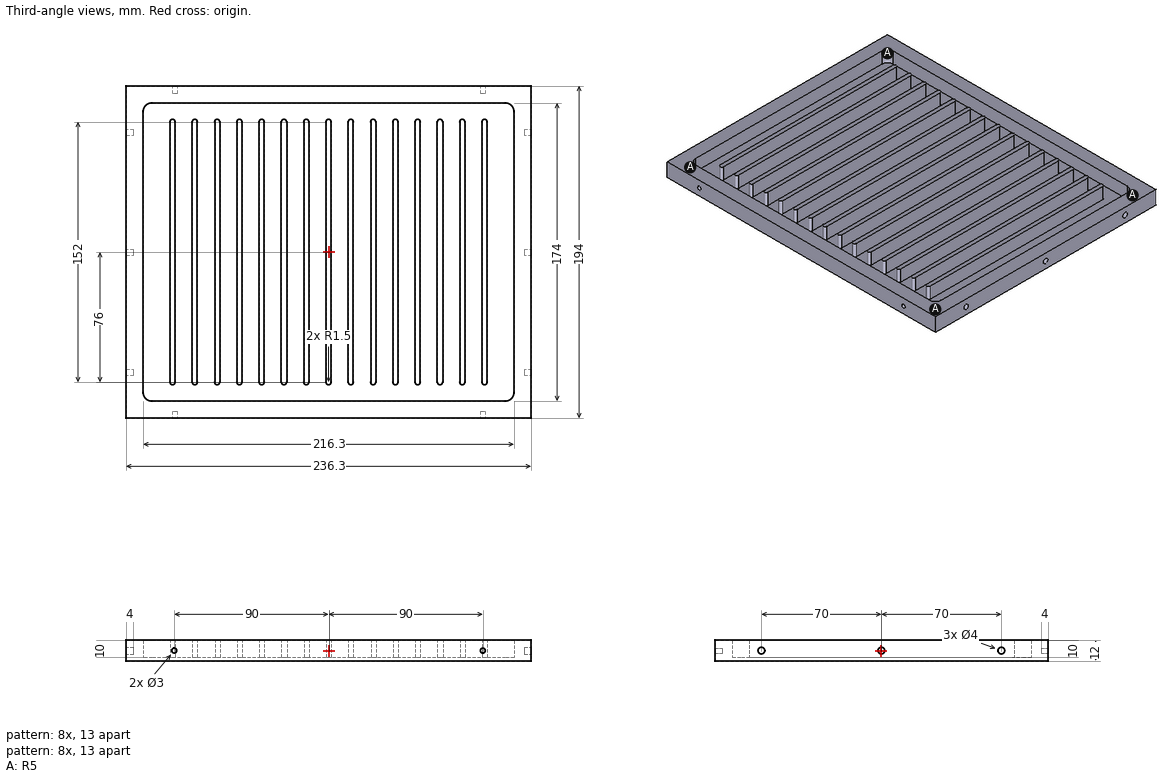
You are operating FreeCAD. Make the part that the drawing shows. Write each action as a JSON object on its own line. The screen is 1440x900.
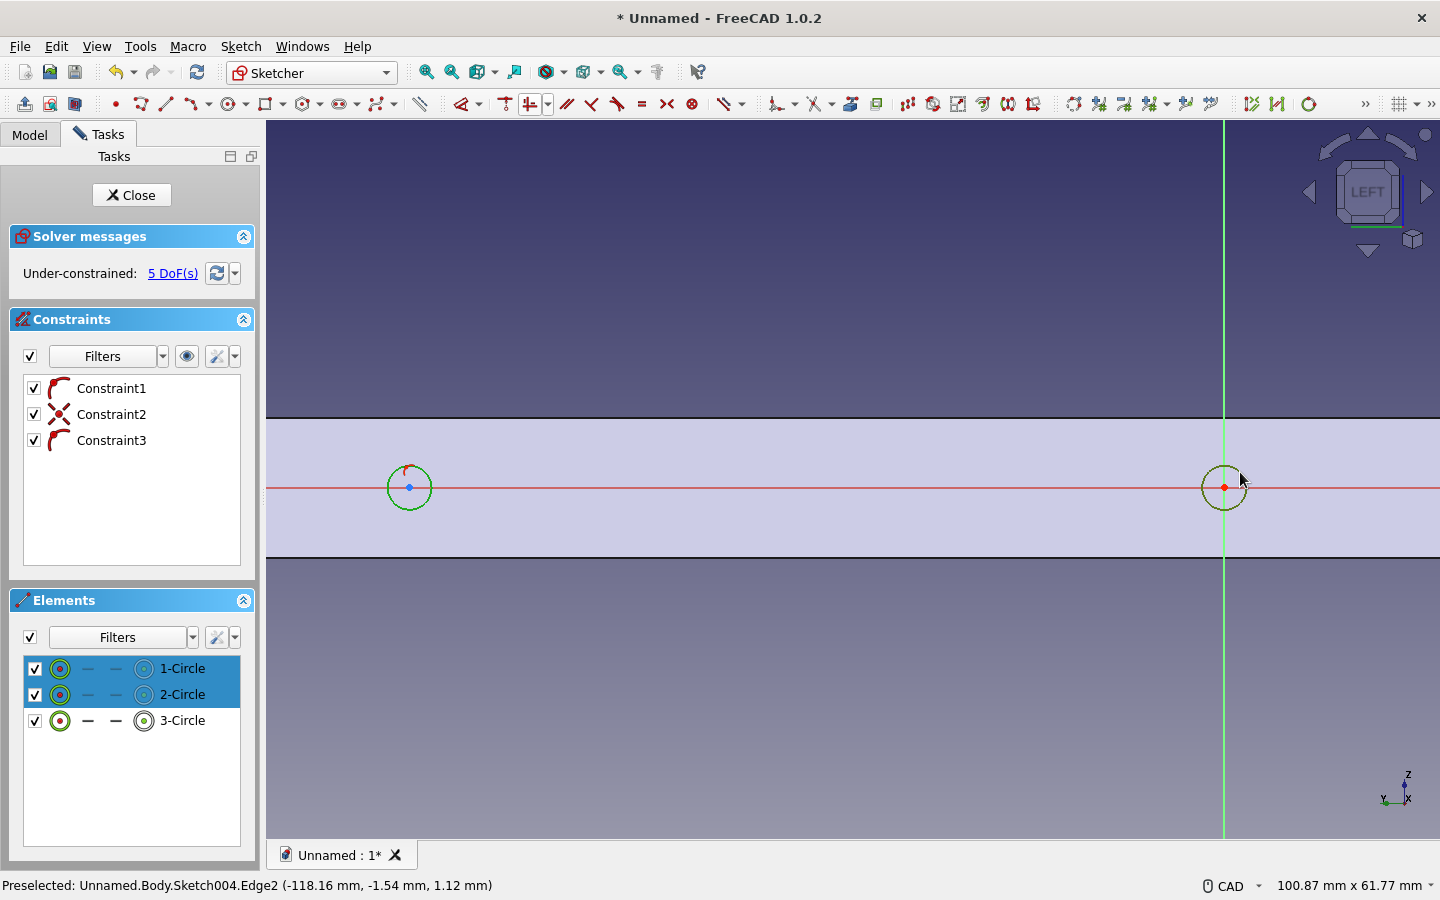
{"action": "scroll", "coordinate": [426, 473], "scroll_direction": "down", "scroll_amount": 4}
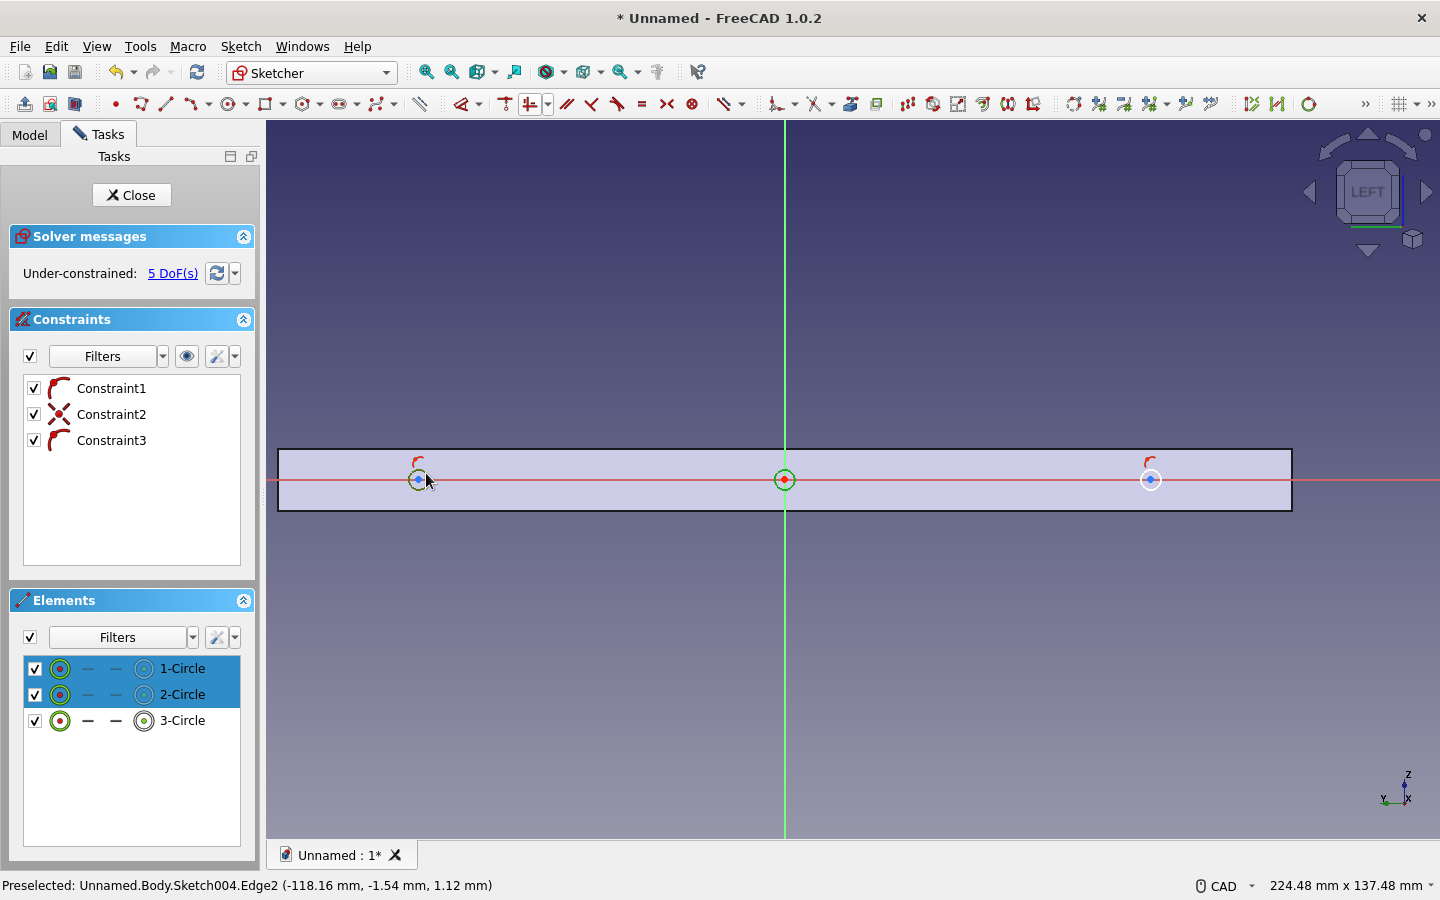
{"action": "scroll", "coordinate": [1158, 473], "scroll_direction": "up", "scroll_amount": 4}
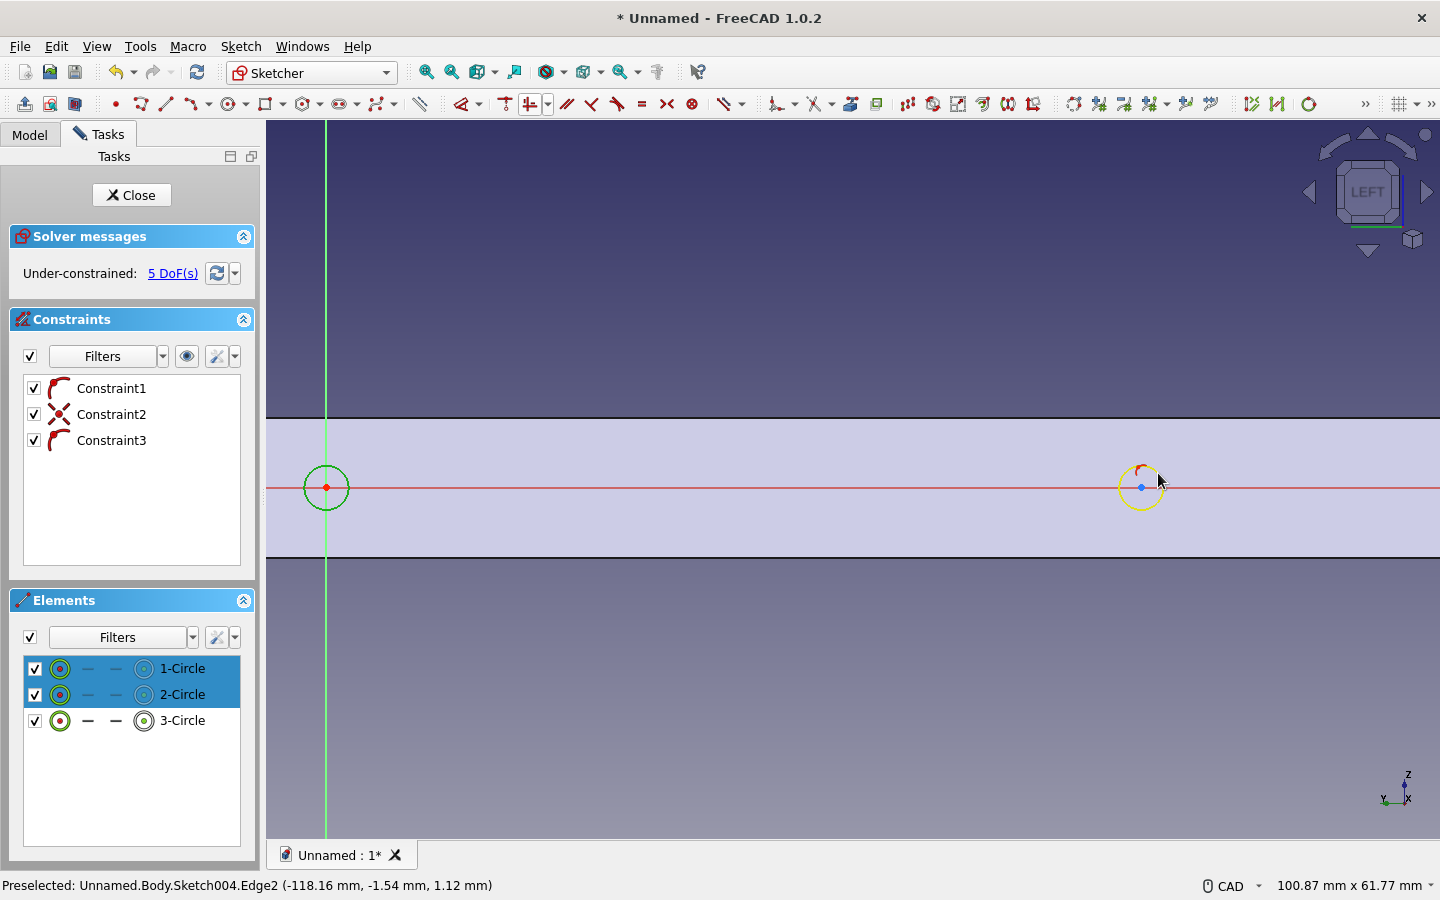
{"action": "left_click", "coordinate": [1157, 472]}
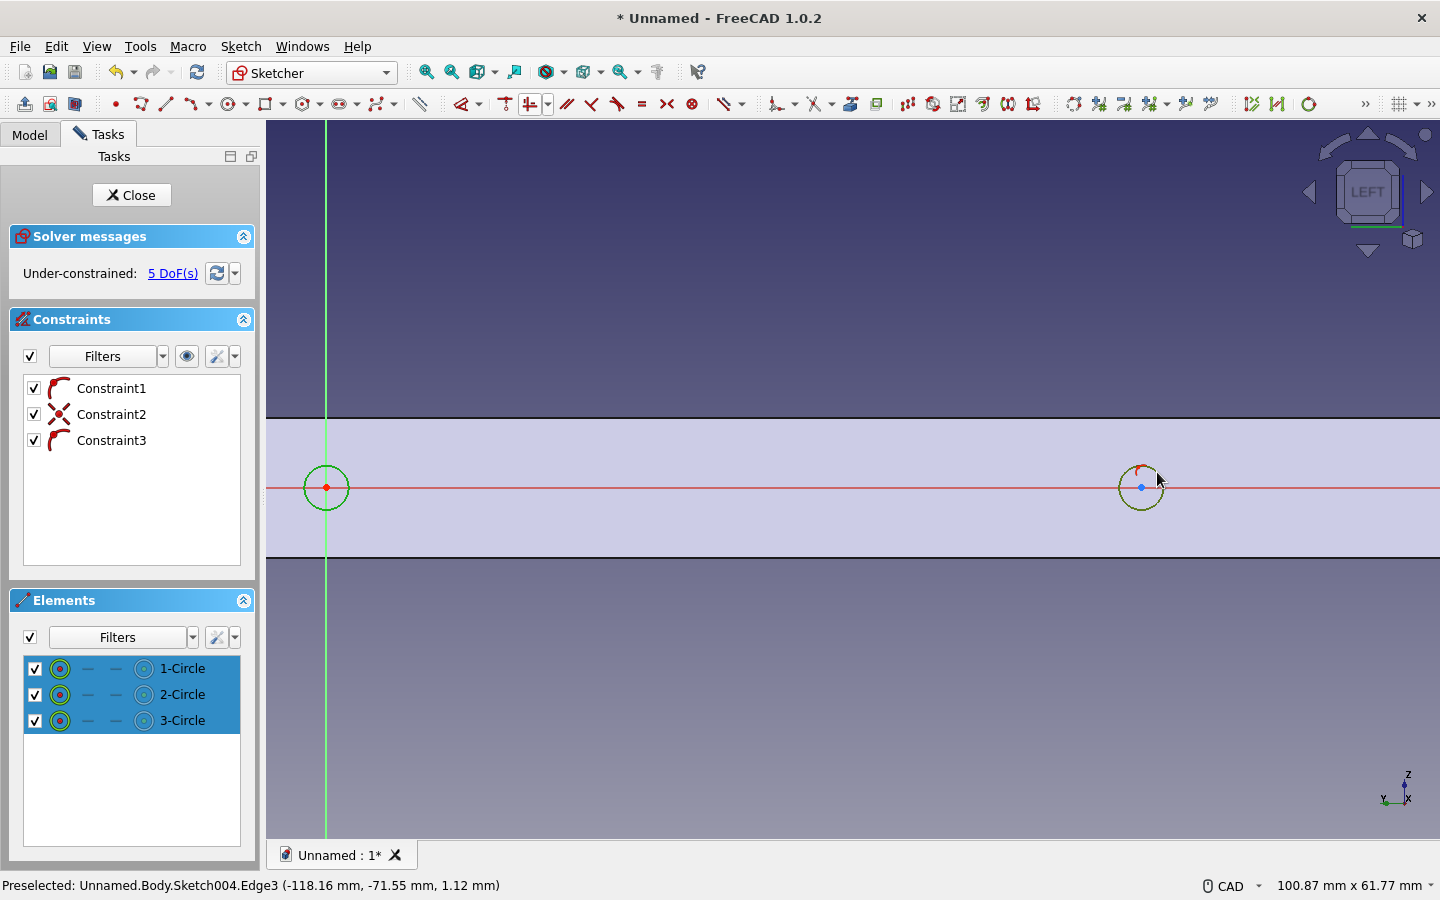
{"action": "left_click", "coordinate": [642, 104]}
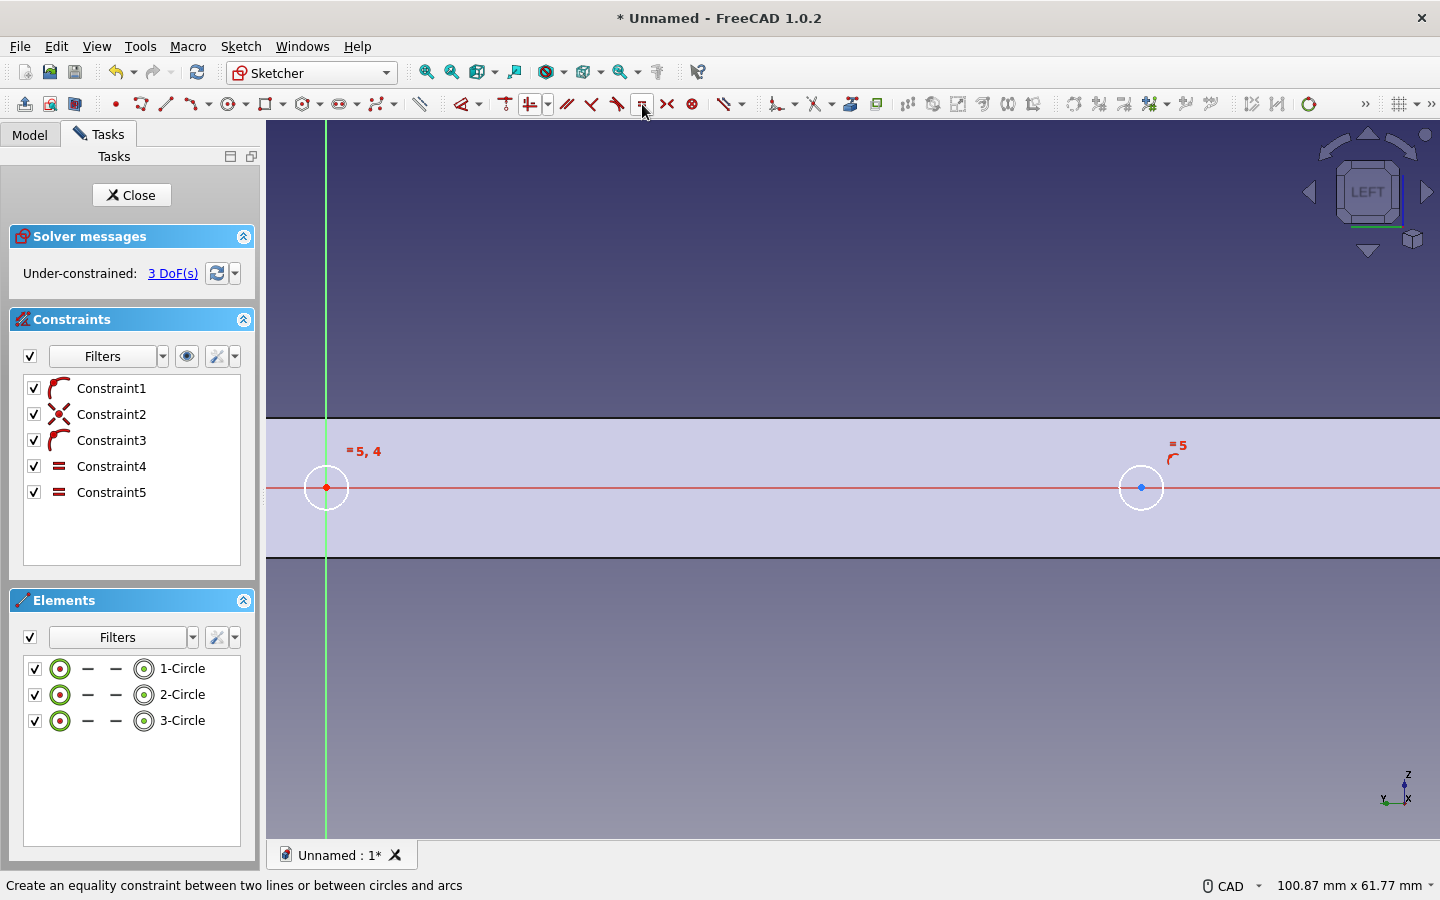
{"action": "left_click", "coordinate": [460, 104]}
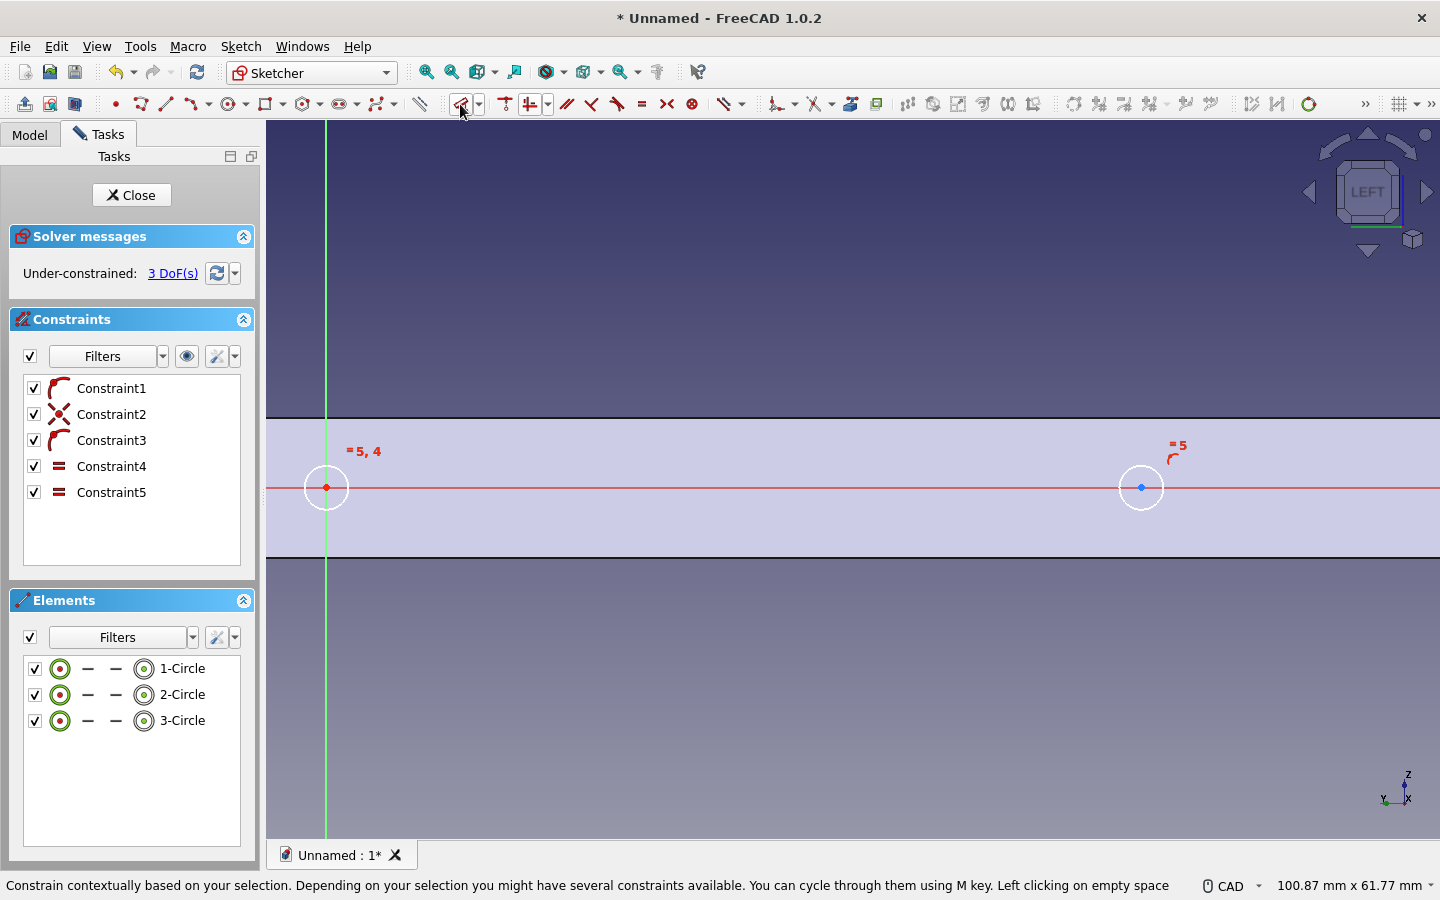
{"action": "scroll", "coordinate": [1158, 473], "scroll_direction": "down", "scroll_amount": 4}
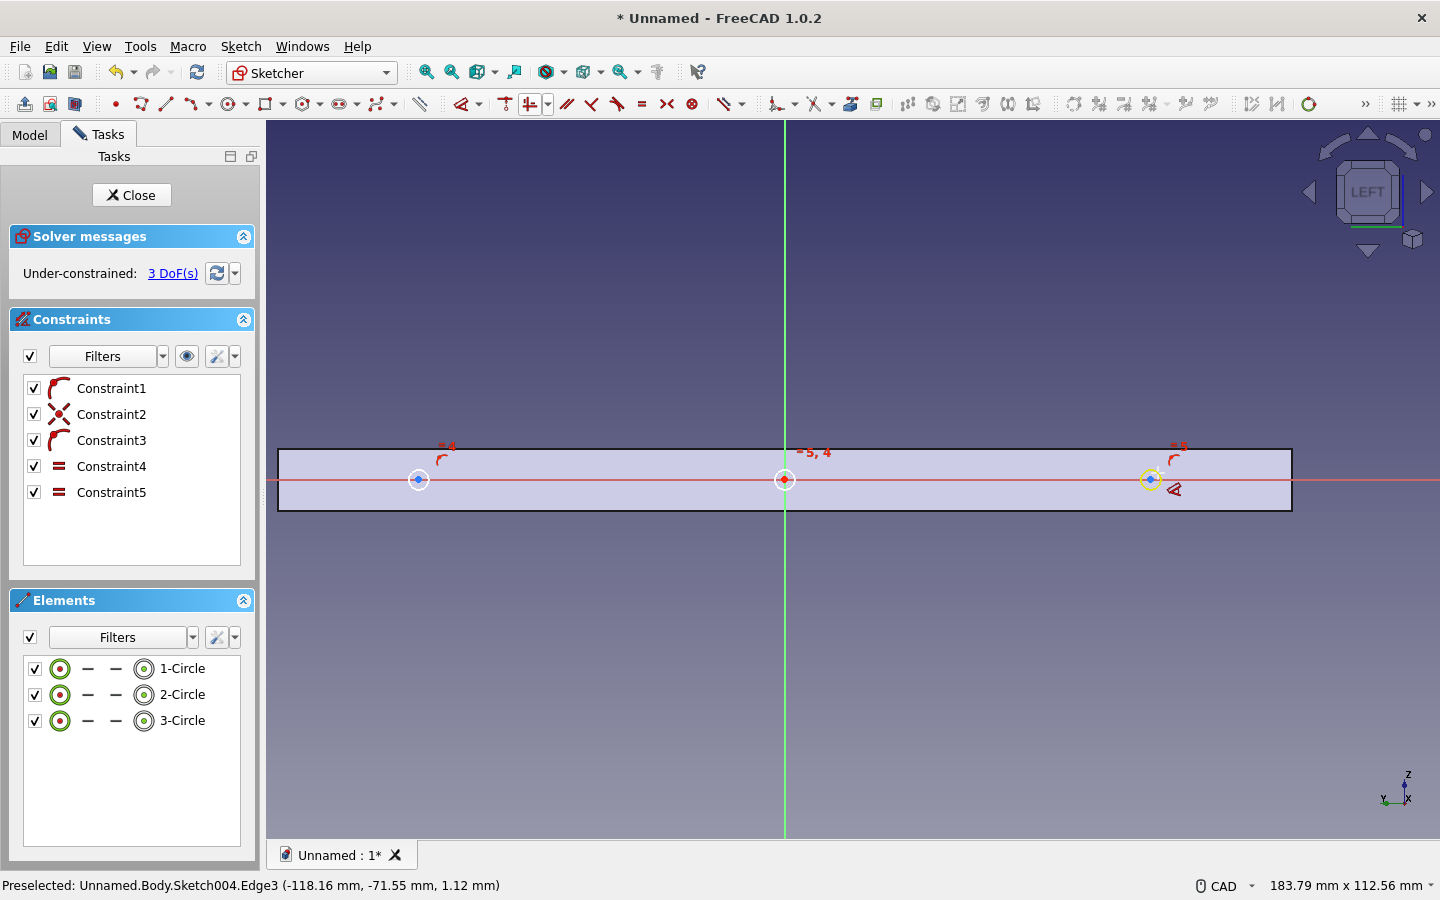
{"action": "scroll", "coordinate": [426, 473], "scroll_direction": "up", "scroll_amount": 4}